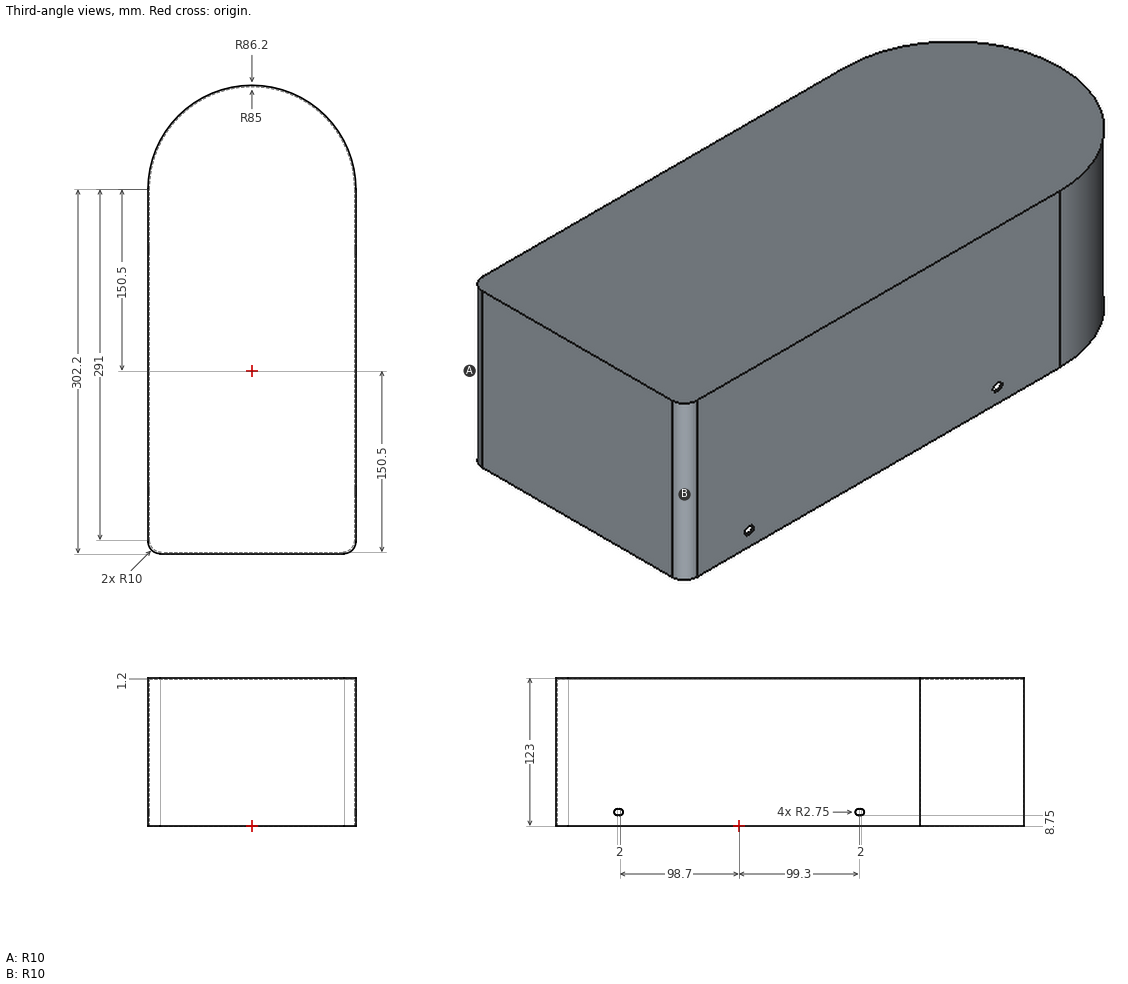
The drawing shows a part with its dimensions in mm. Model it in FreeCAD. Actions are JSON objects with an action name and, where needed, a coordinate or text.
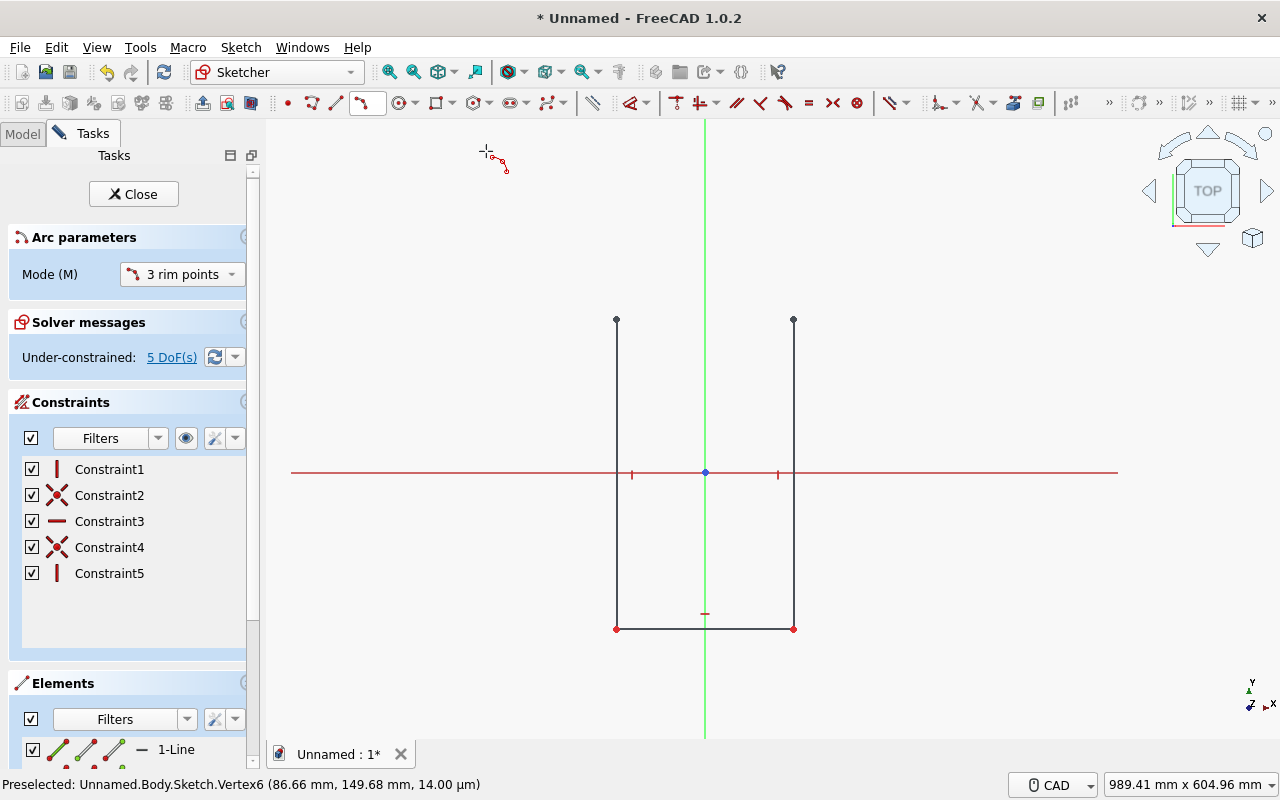
{"action": "left_click", "coordinate": [794, 319]}
{"action": "left_click", "coordinate": [617, 319]}
{"action": "left_click", "coordinate": [732, 234]}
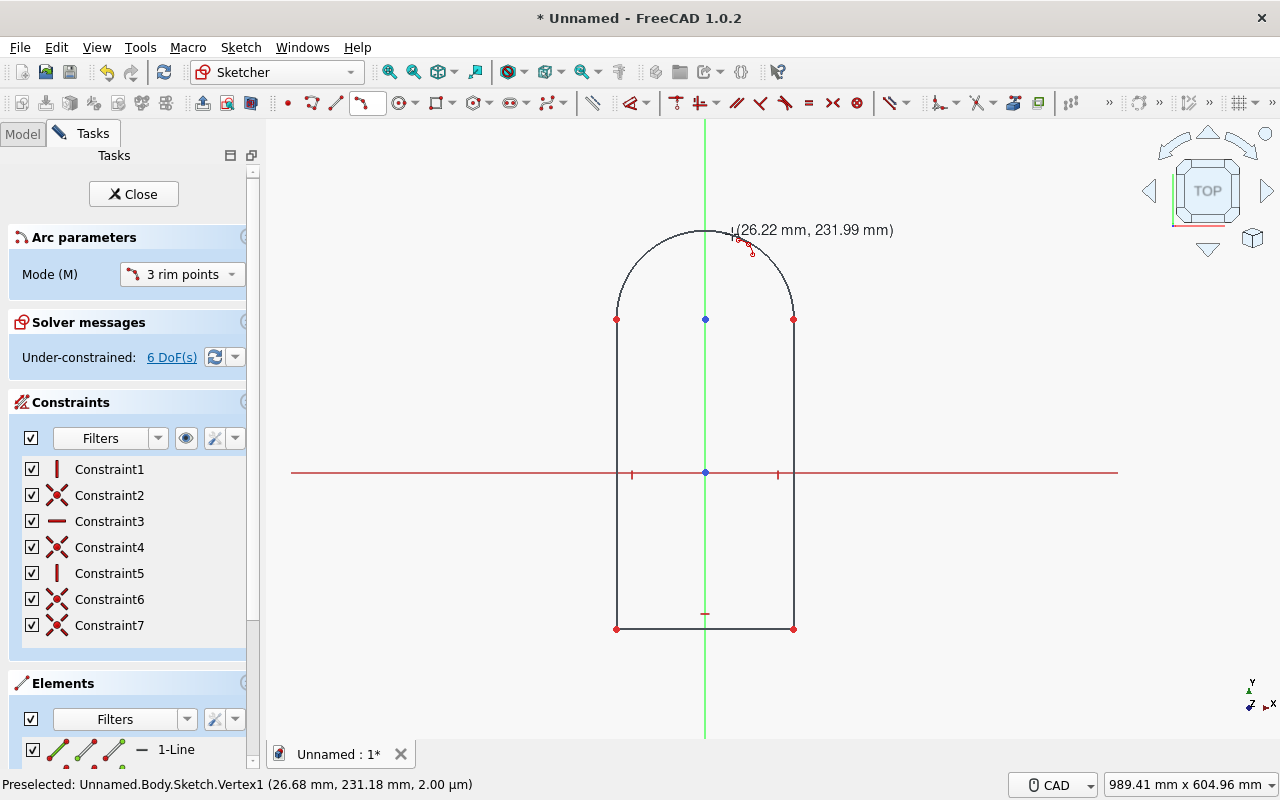
{"action": "left_click", "coordinate": [336, 104]}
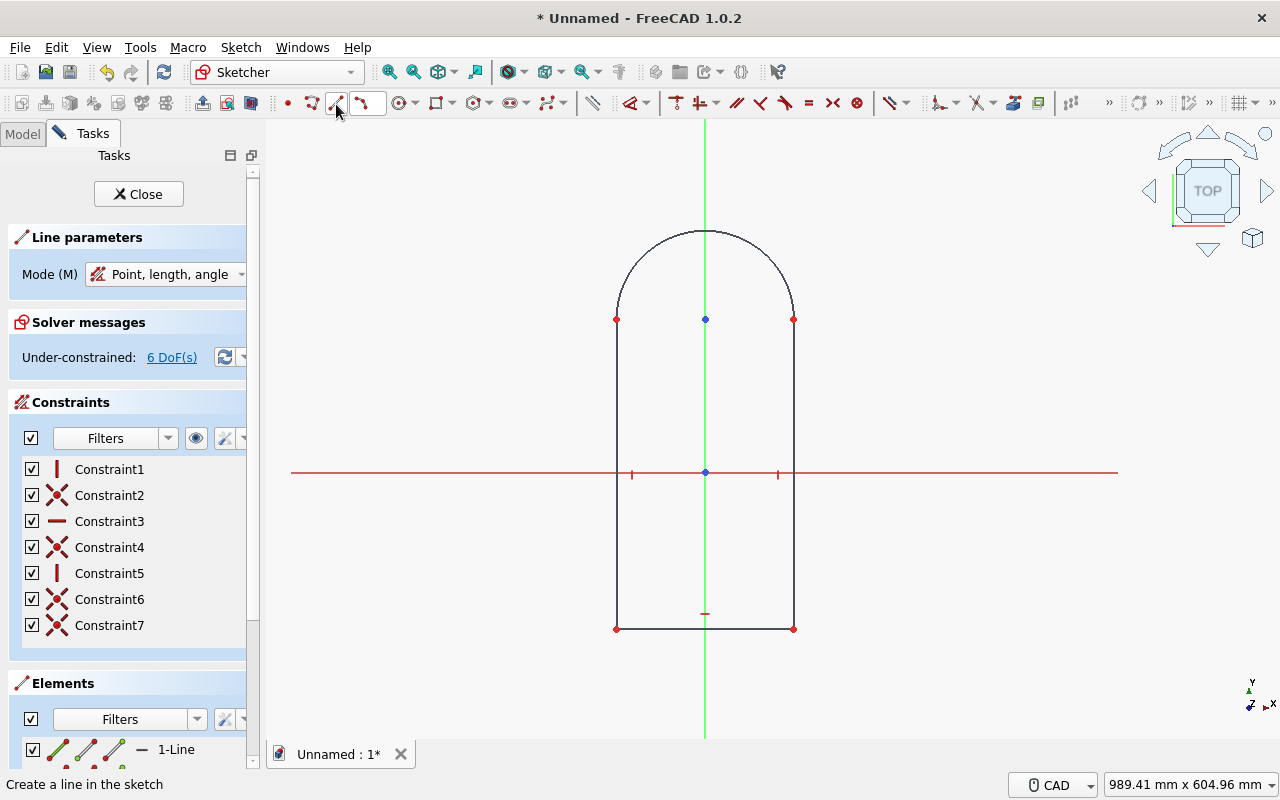
{"action": "scroll", "coordinate": [782, 627], "scroll_direction": "up", "scroll_amount": 13}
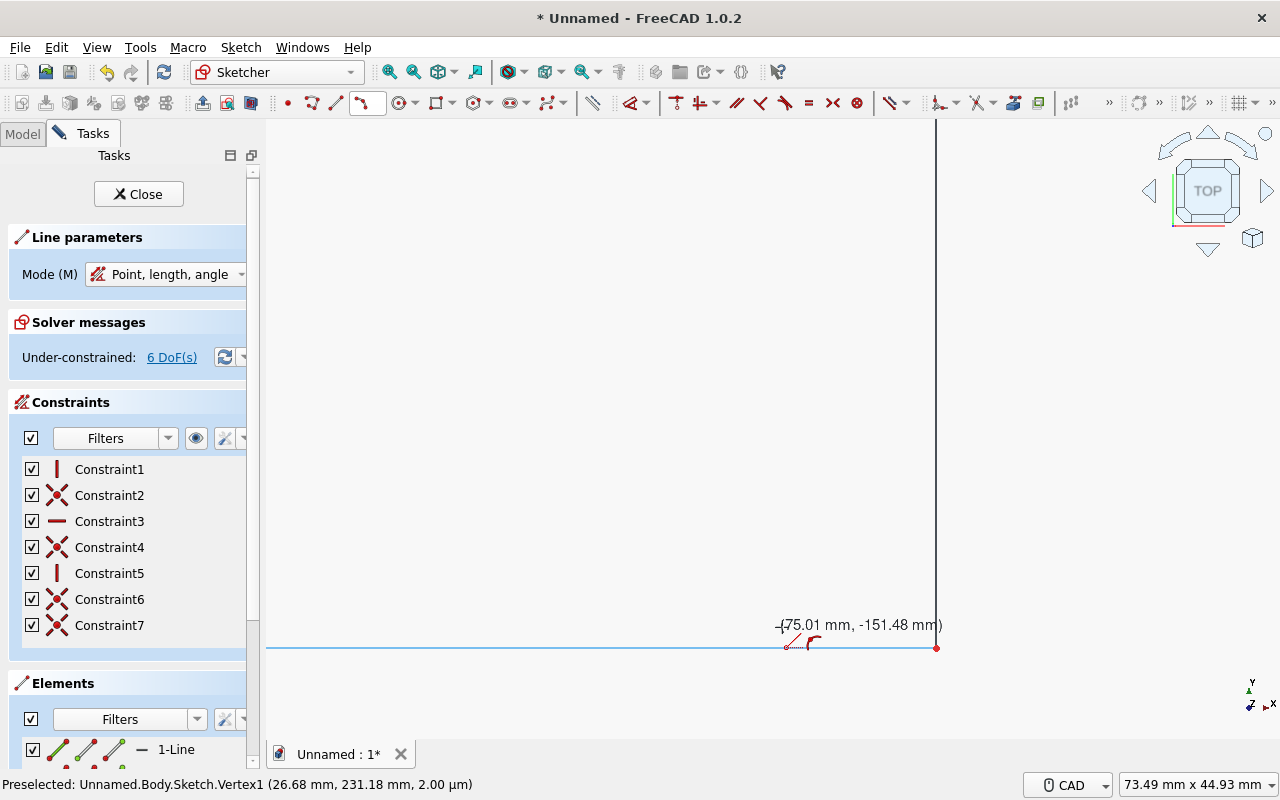
{"action": "left_click", "coordinate": [775, 617]}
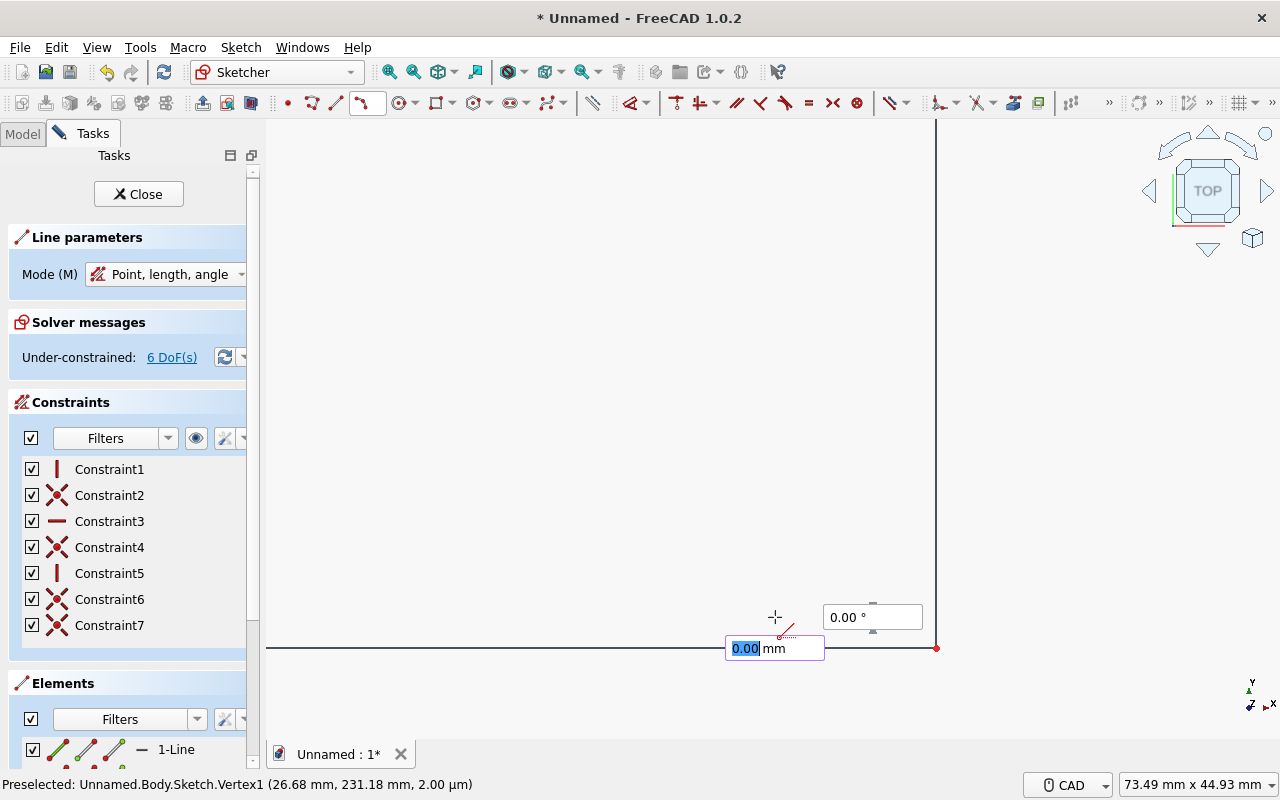
{"action": "scroll", "coordinate": [782, 628], "scroll_direction": "down", "scroll_amount": 13}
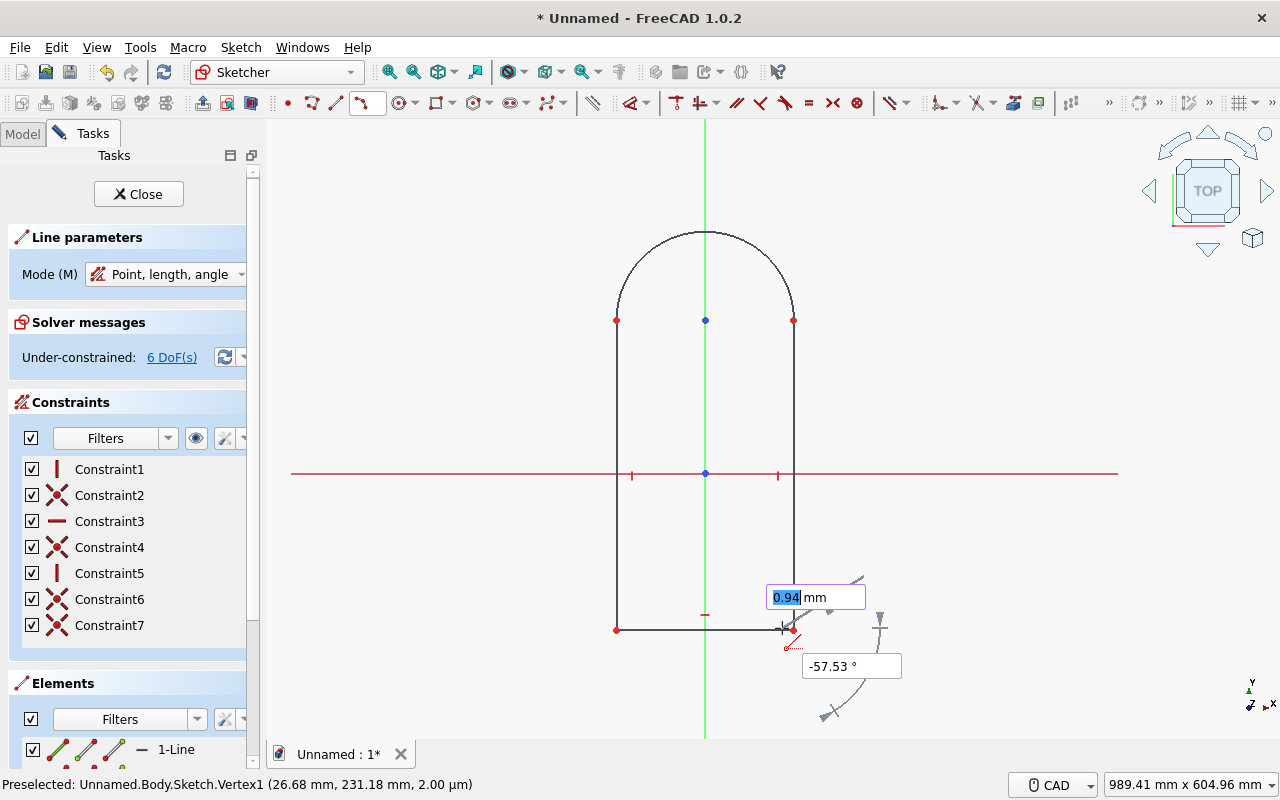
{"action": "scroll", "coordinate": [628, 628], "scroll_direction": "up", "scroll_amount": 13}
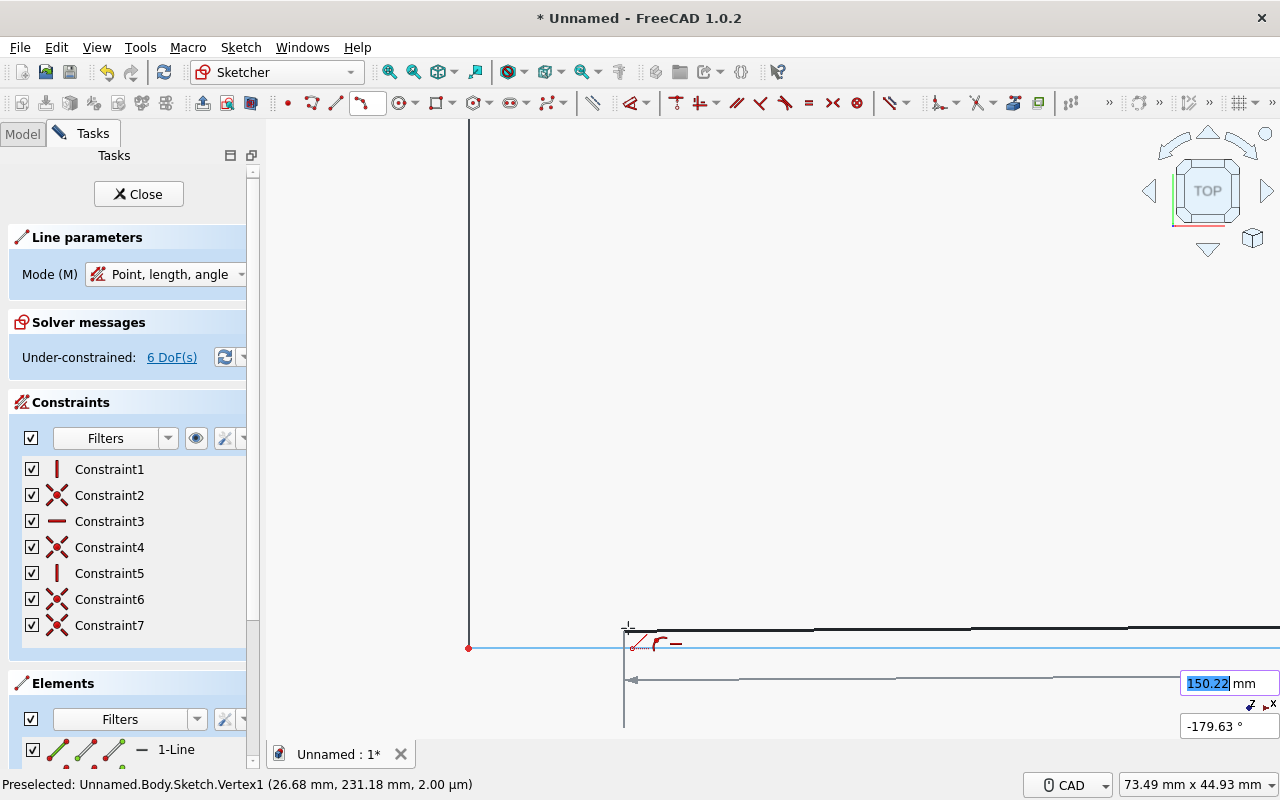
{"action": "left_click", "coordinate": [627, 617]}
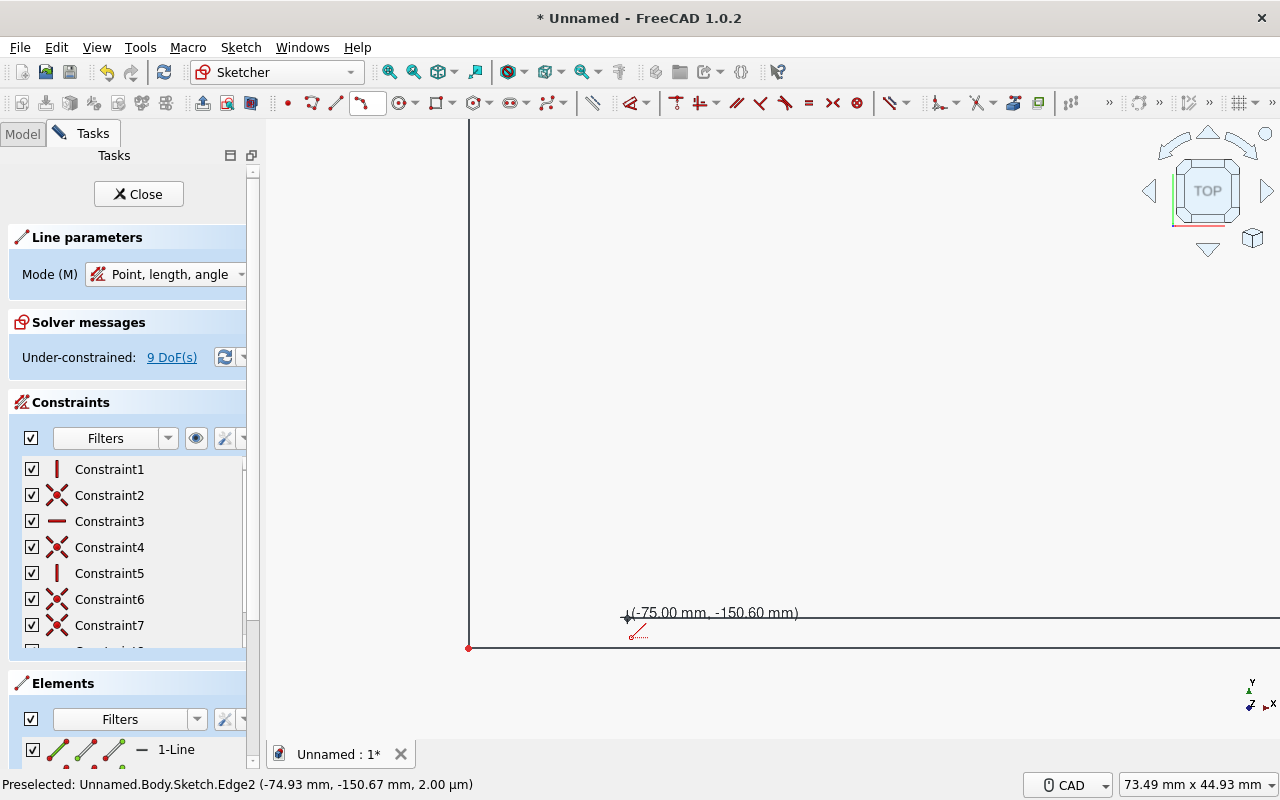
{"action": "left_click", "coordinate": [489, 479]}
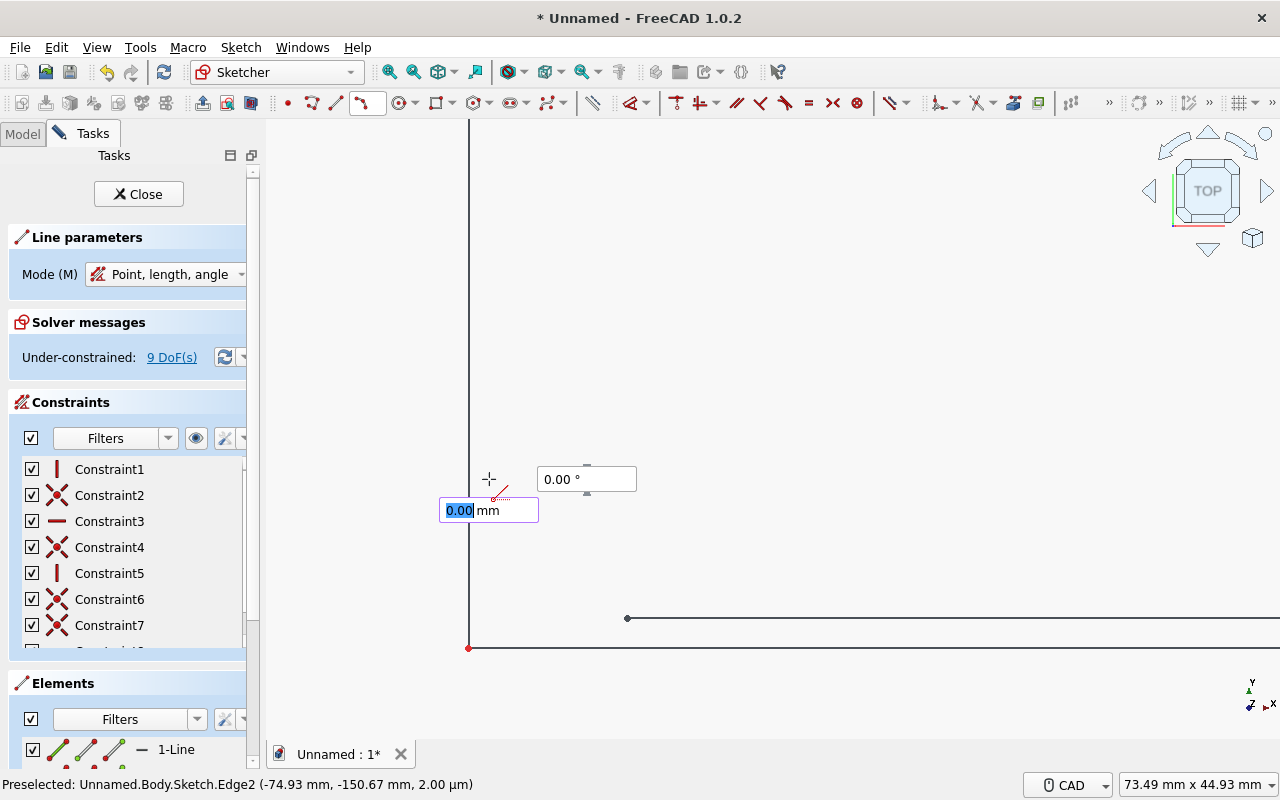
{"action": "scroll", "coordinate": [628, 628], "scroll_direction": "down", "scroll_amount": 13}